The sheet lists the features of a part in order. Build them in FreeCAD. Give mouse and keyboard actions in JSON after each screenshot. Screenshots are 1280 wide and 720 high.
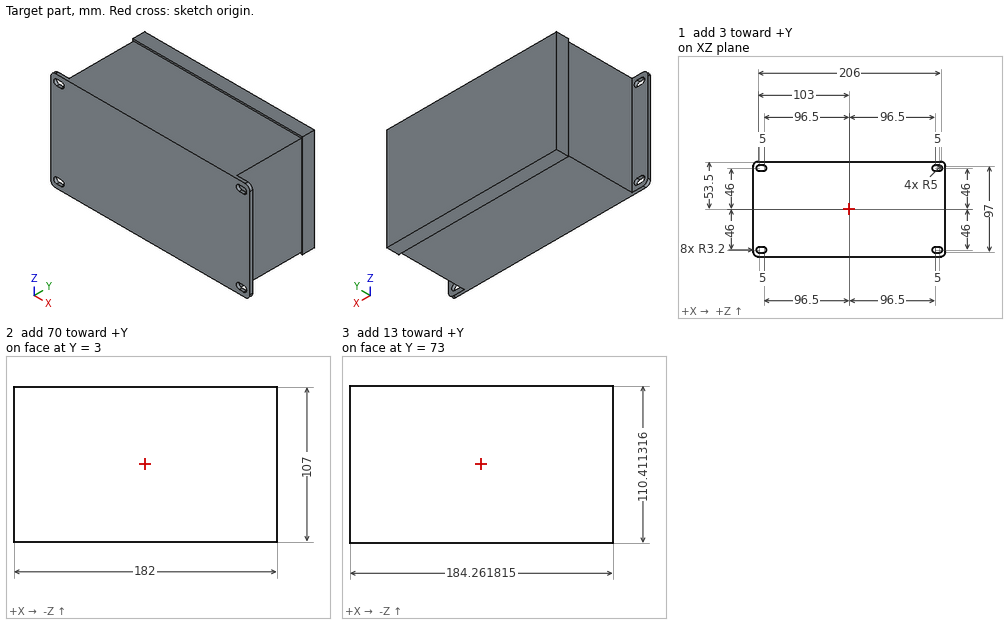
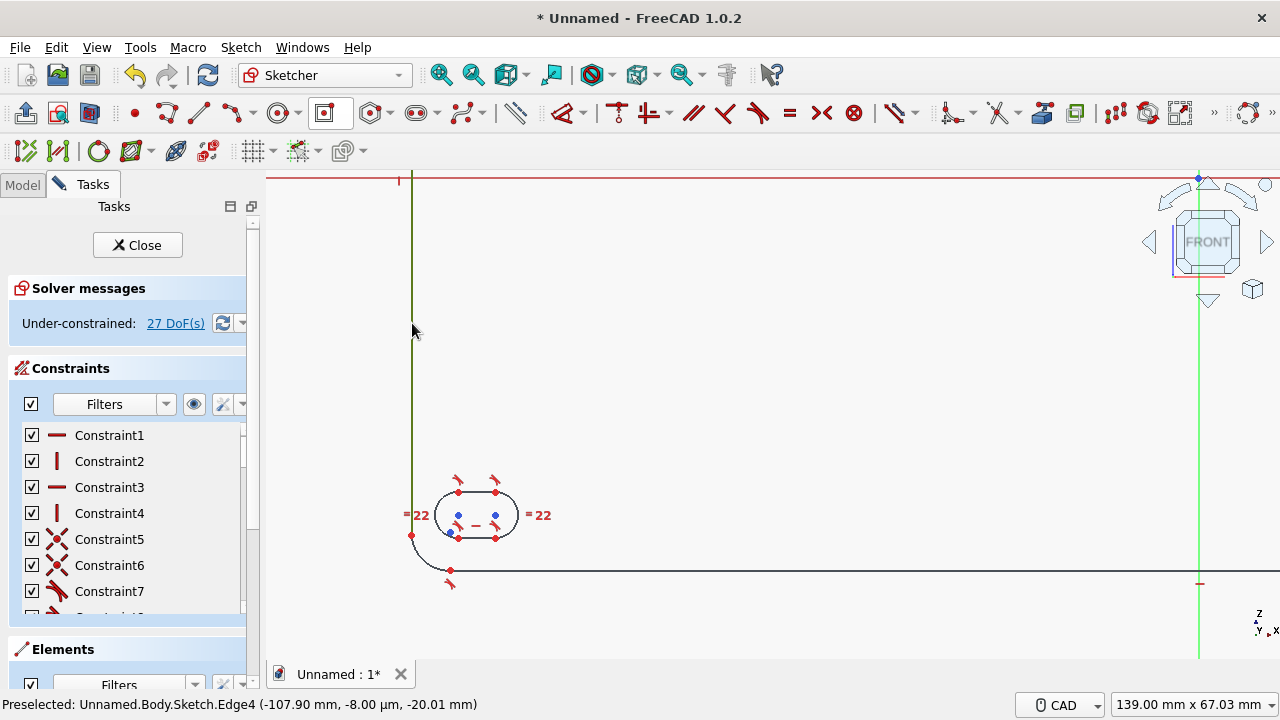
{"action": "left_click", "coordinate": [417, 552]}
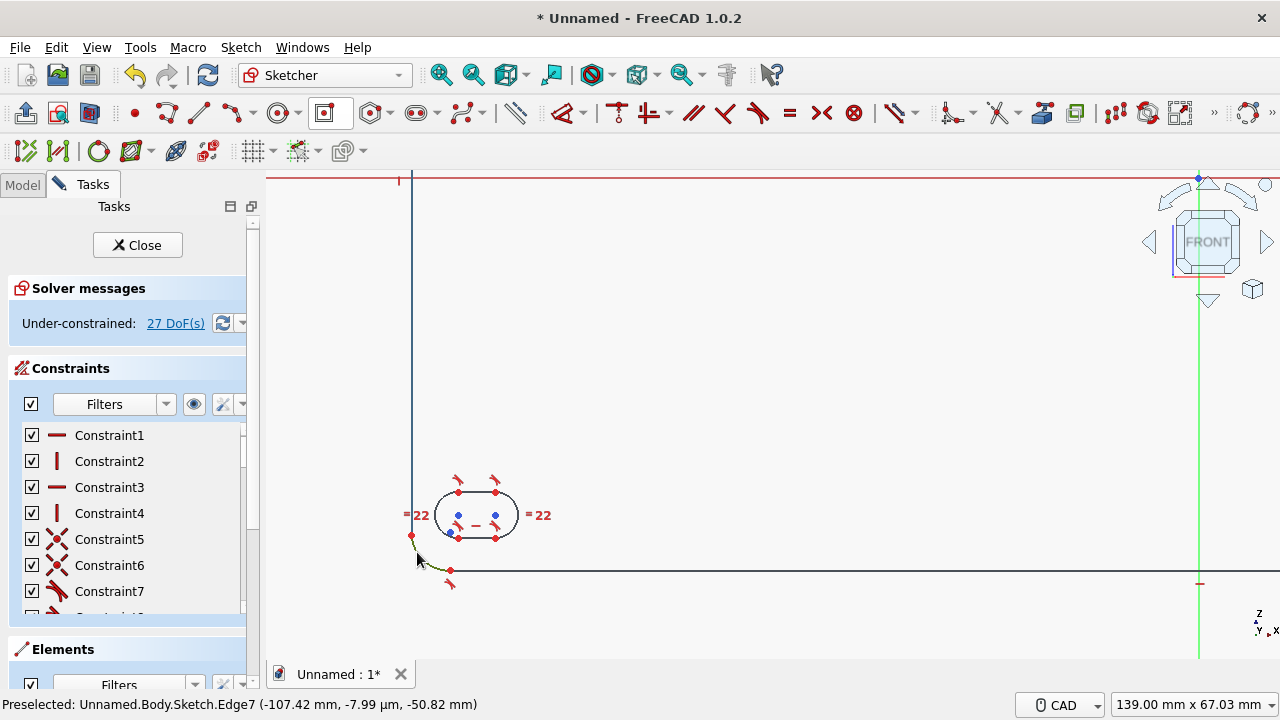
{"action": "left_click", "coordinate": [758, 114]}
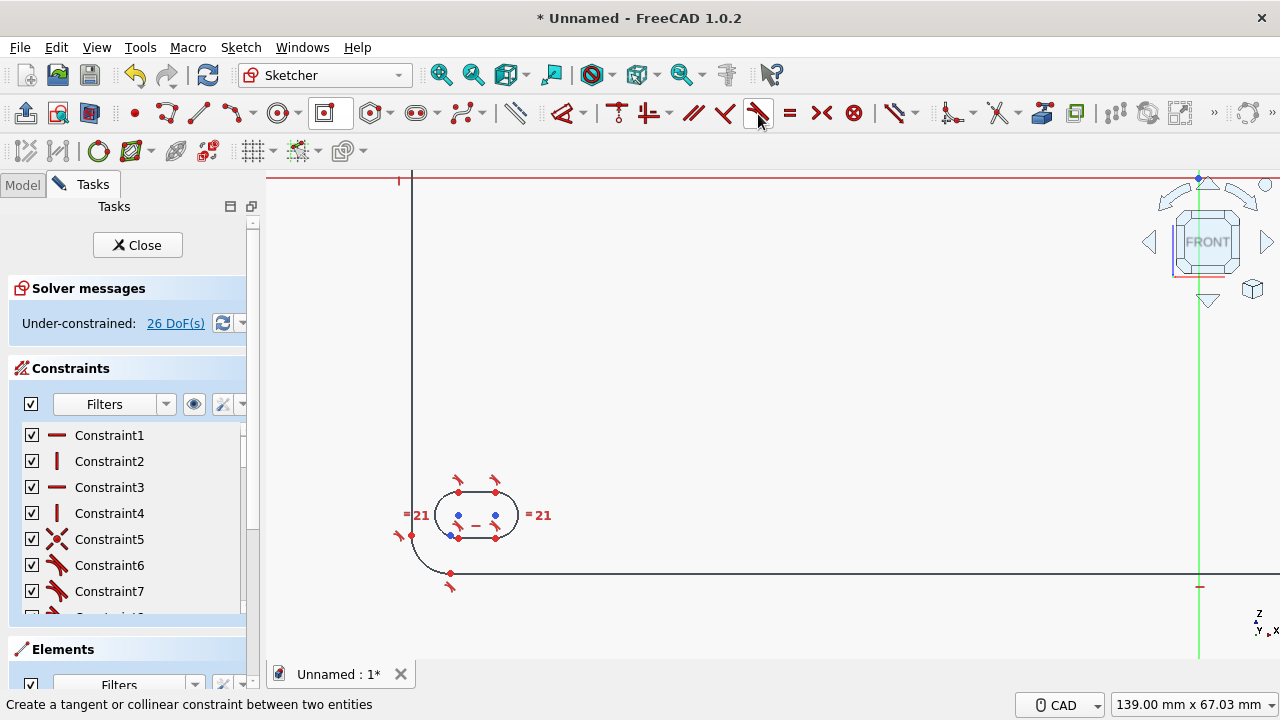
{"action": "left_click", "coordinate": [412, 323]}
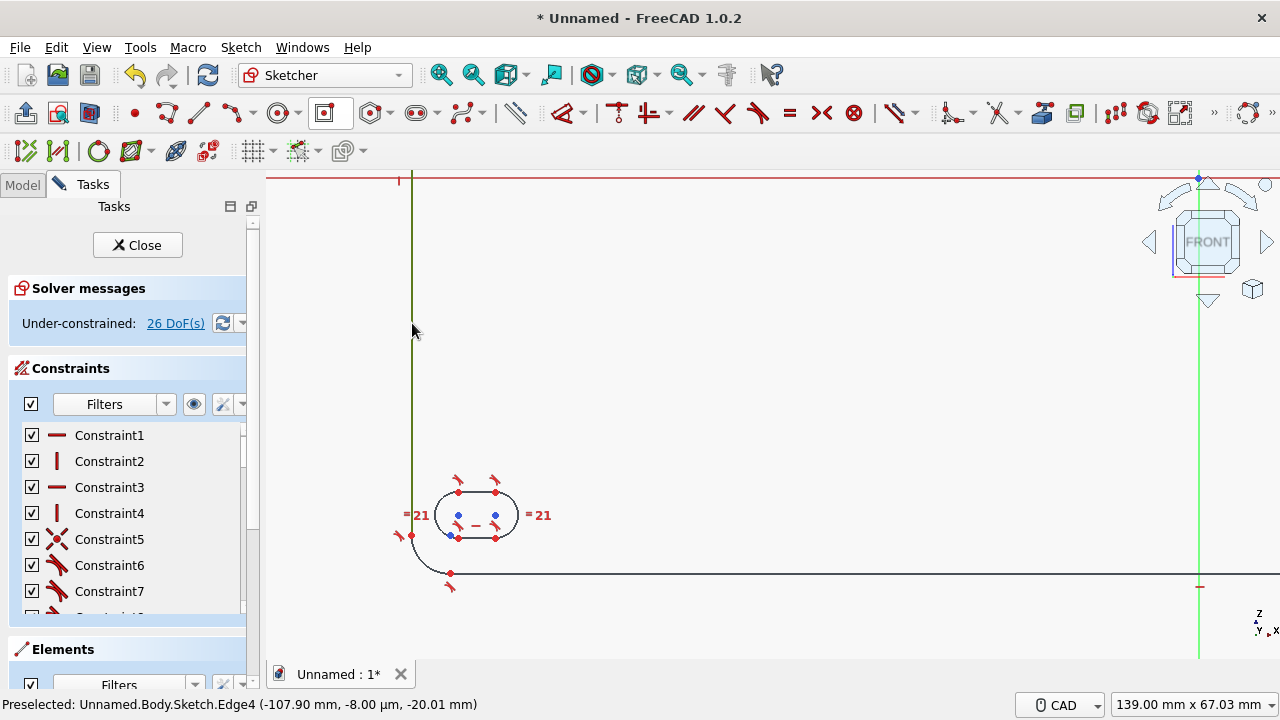
{"action": "scroll", "coordinate": [417, 552], "scroll_direction": "down", "scroll_amount": 5}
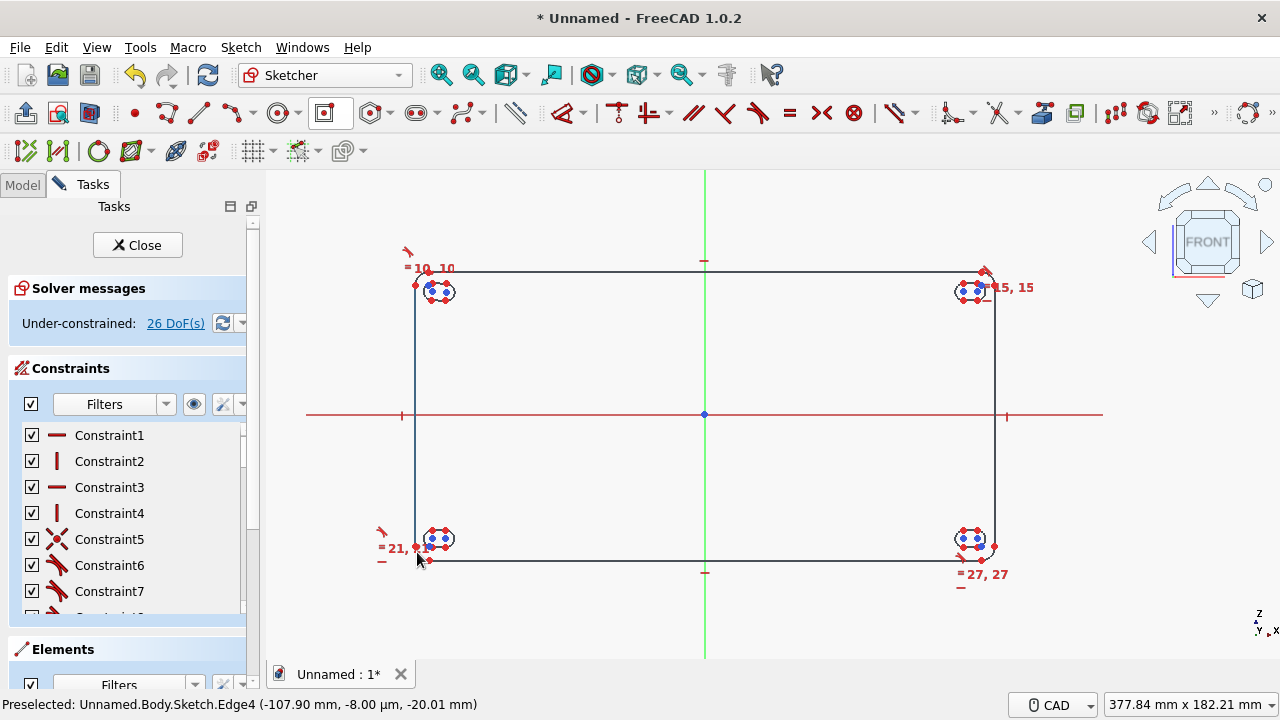
{"action": "scroll", "coordinate": [422, 274], "scroll_direction": "up", "scroll_amount": 5}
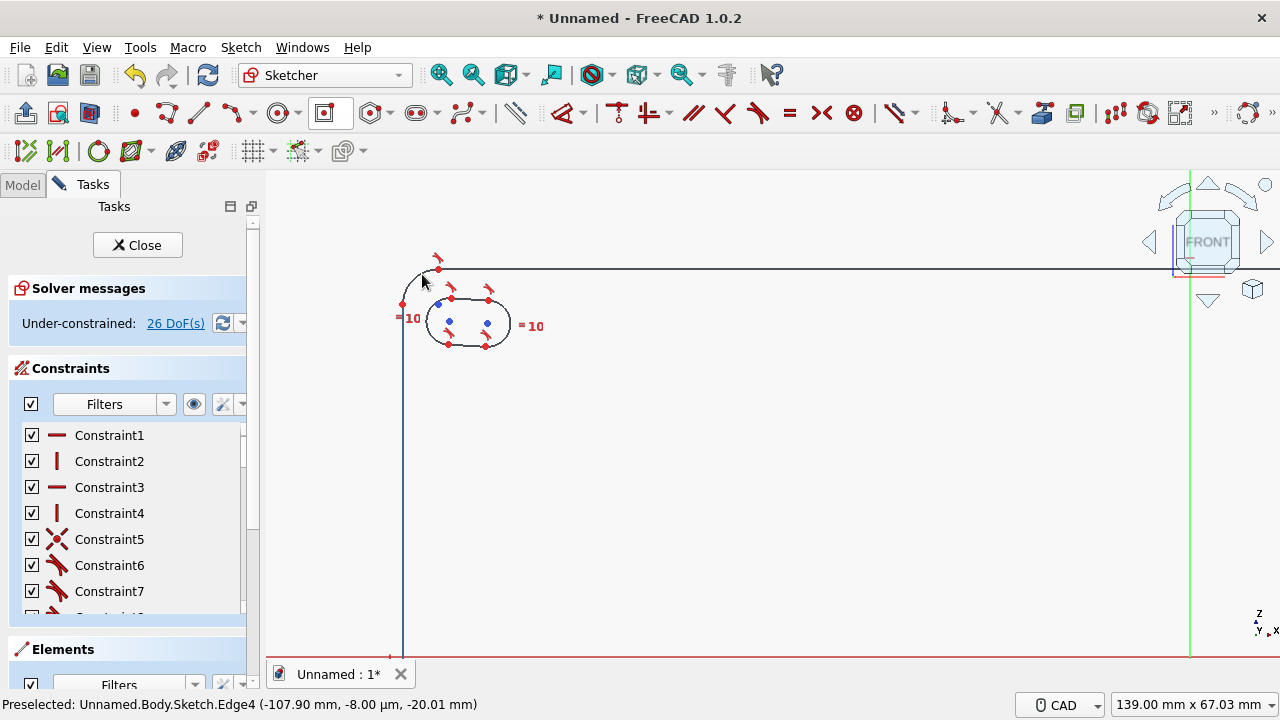
{"action": "left_click", "coordinate": [422, 273]}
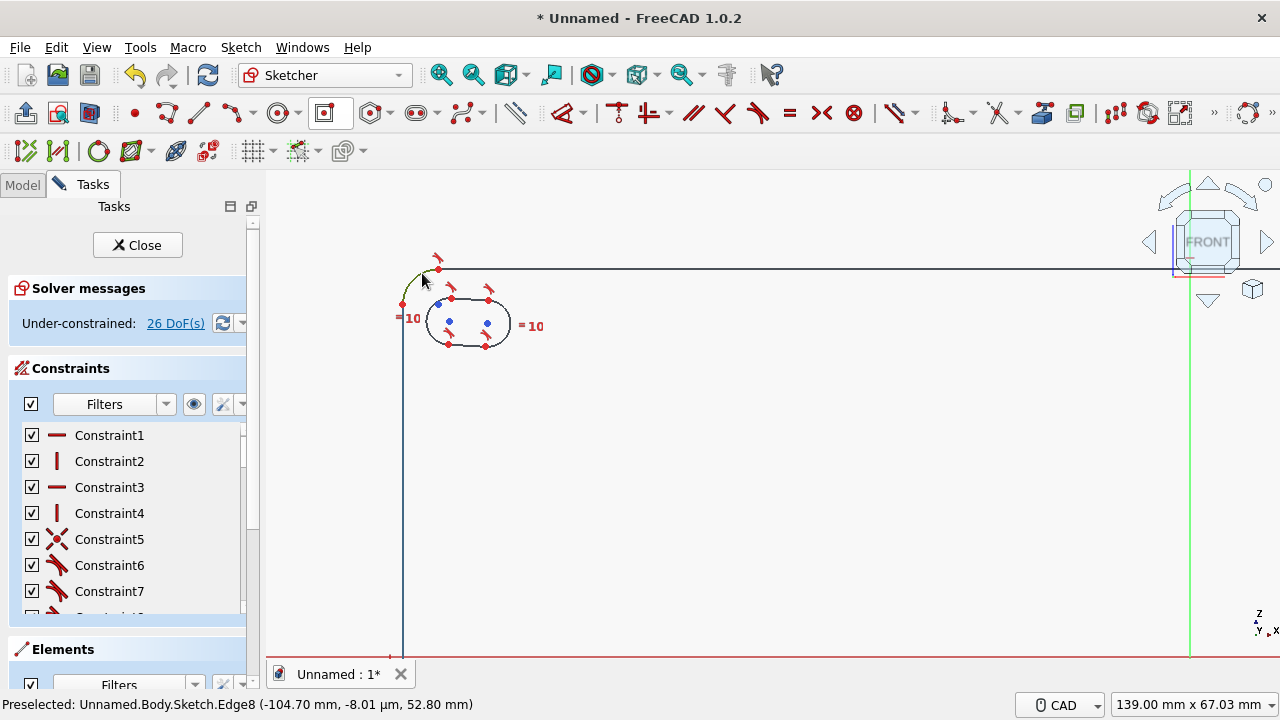
{"action": "left_click", "coordinate": [758, 114]}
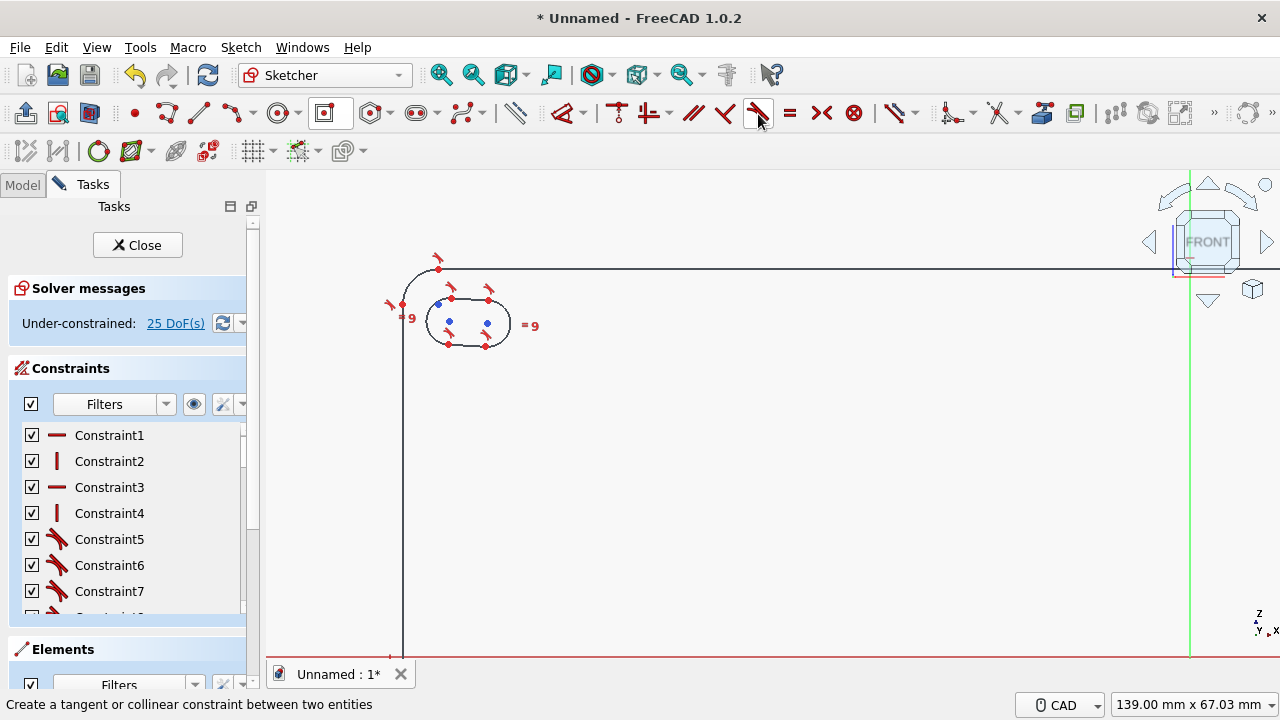
{"action": "scroll", "coordinate": [462, 299], "scroll_direction": "up", "scroll_amount": 2}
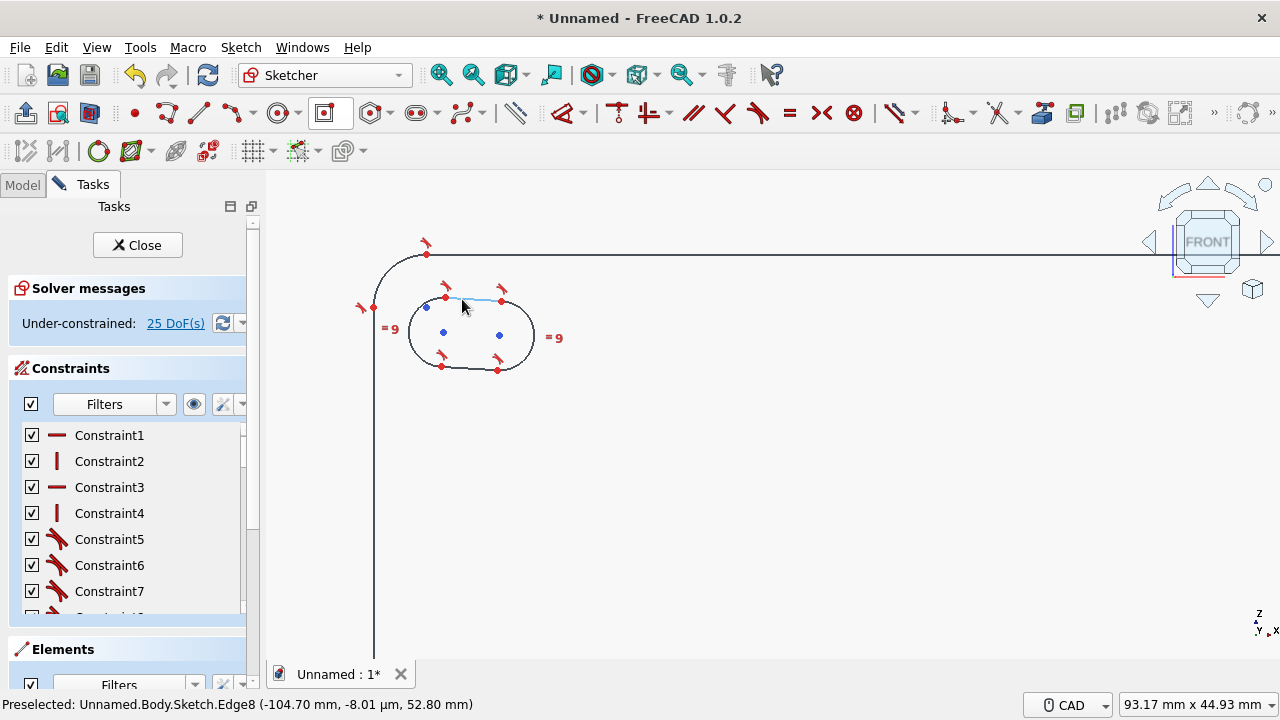
{"action": "left_click", "coordinate": [462, 299]}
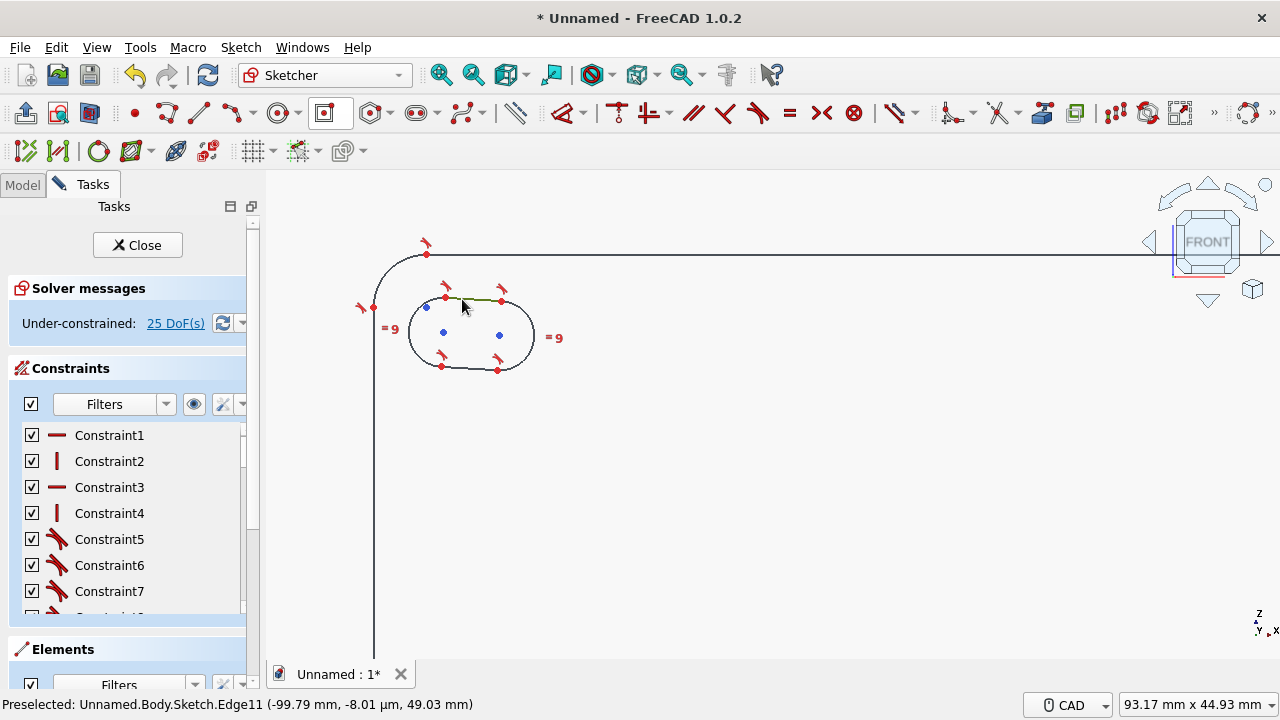
{"action": "key", "text": "h"}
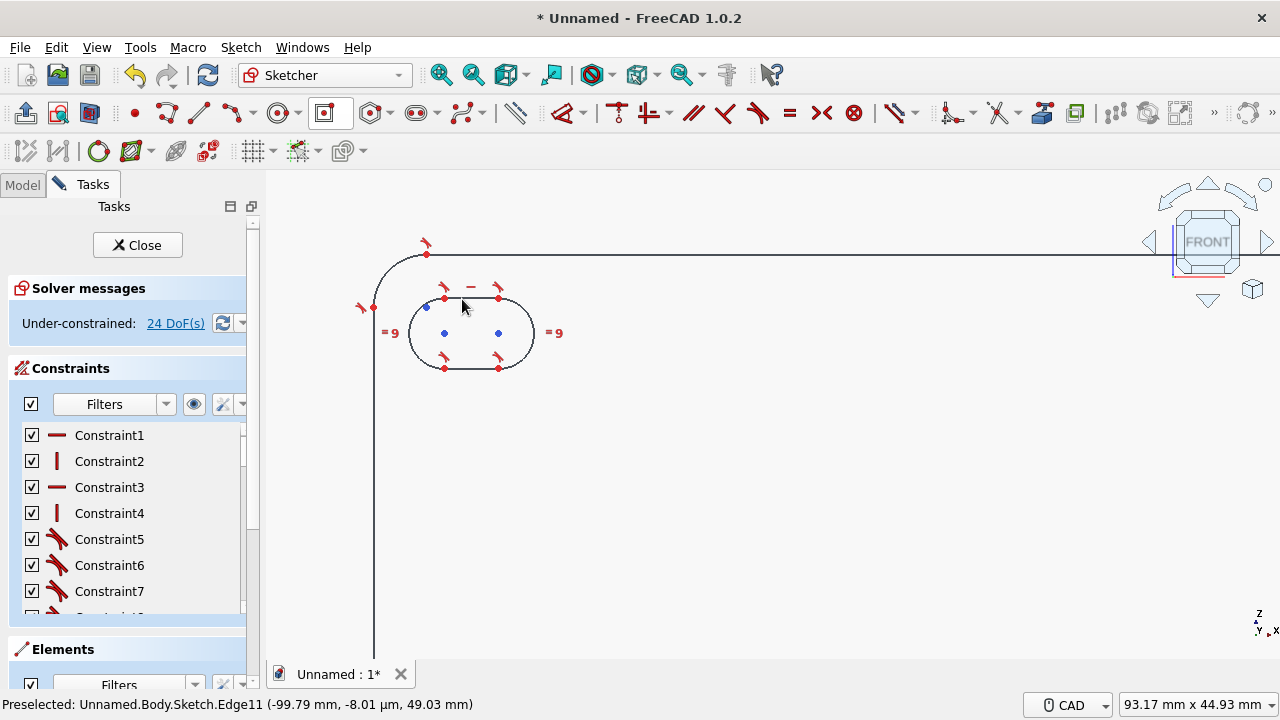
{"action": "scroll", "coordinate": [428, 278], "scroll_direction": "down", "scroll_amount": 7}